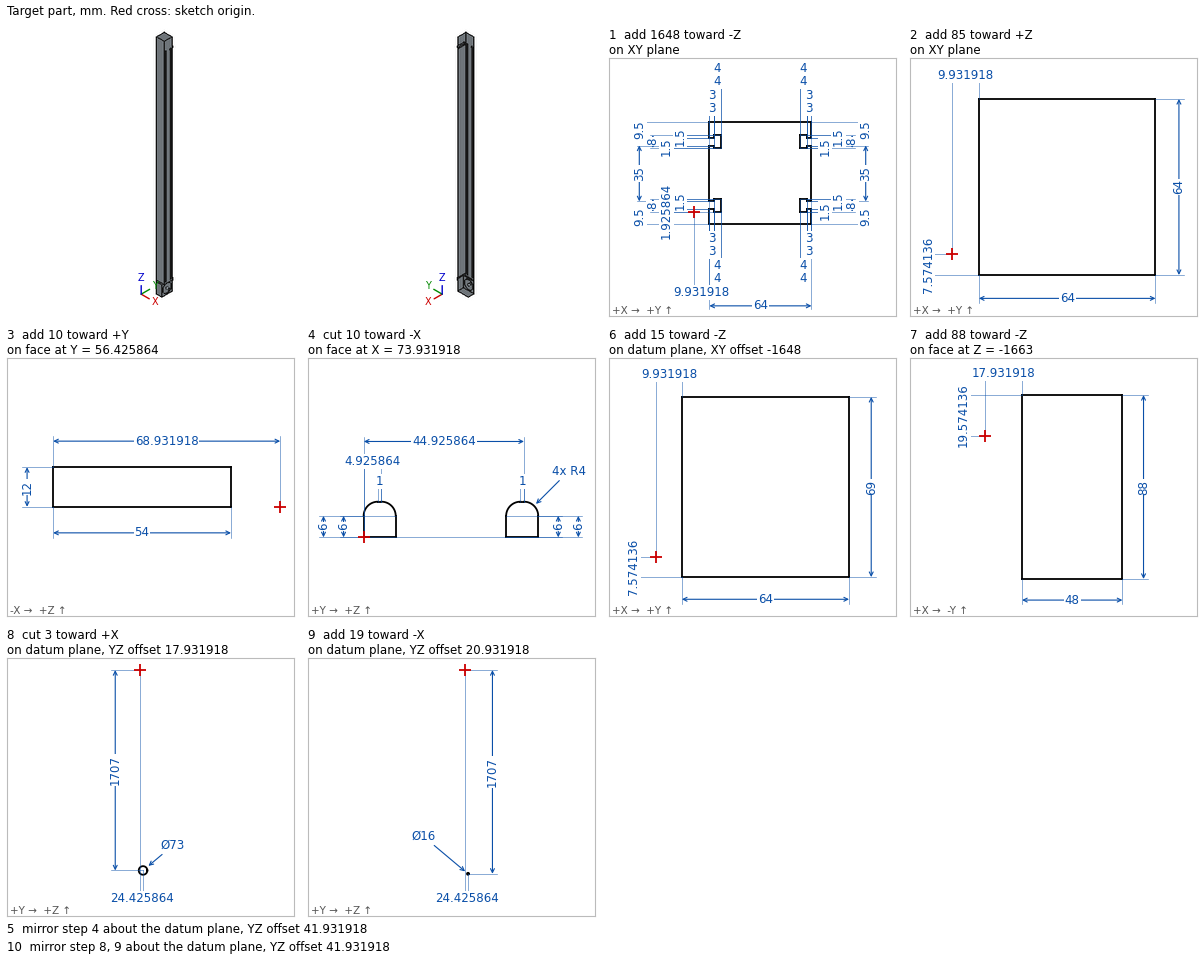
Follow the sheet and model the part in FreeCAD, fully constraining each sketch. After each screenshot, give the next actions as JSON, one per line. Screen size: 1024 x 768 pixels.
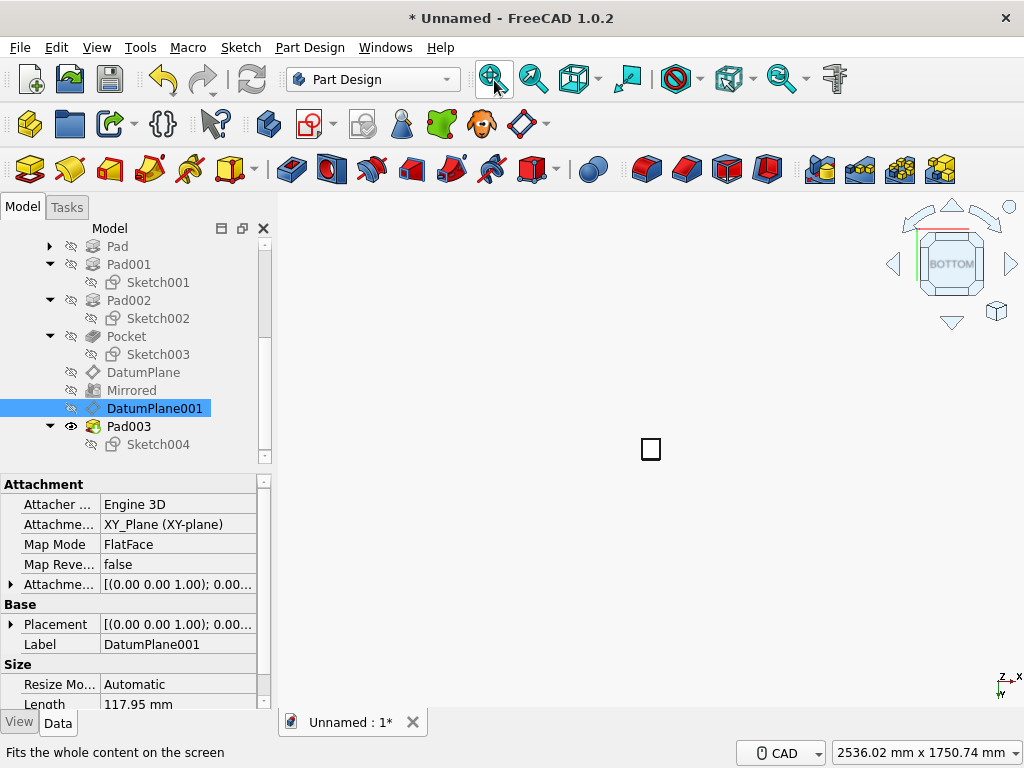
{"action": "left_click", "coordinate": [494, 80]}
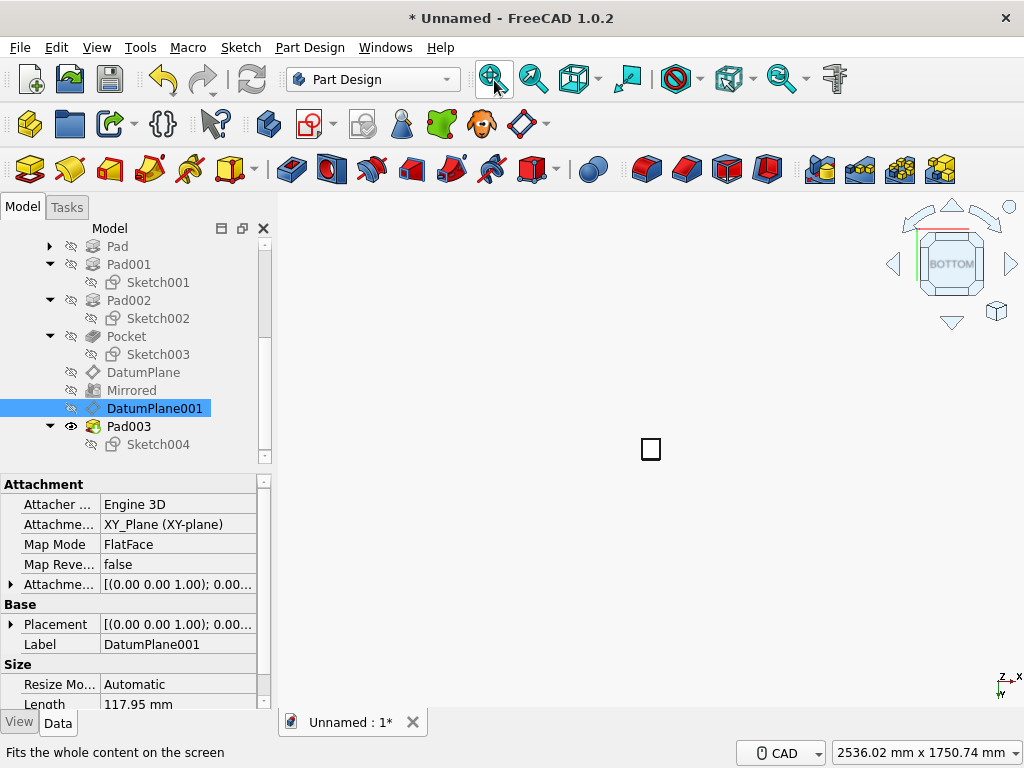
{"action": "left_click", "coordinate": [651, 448]}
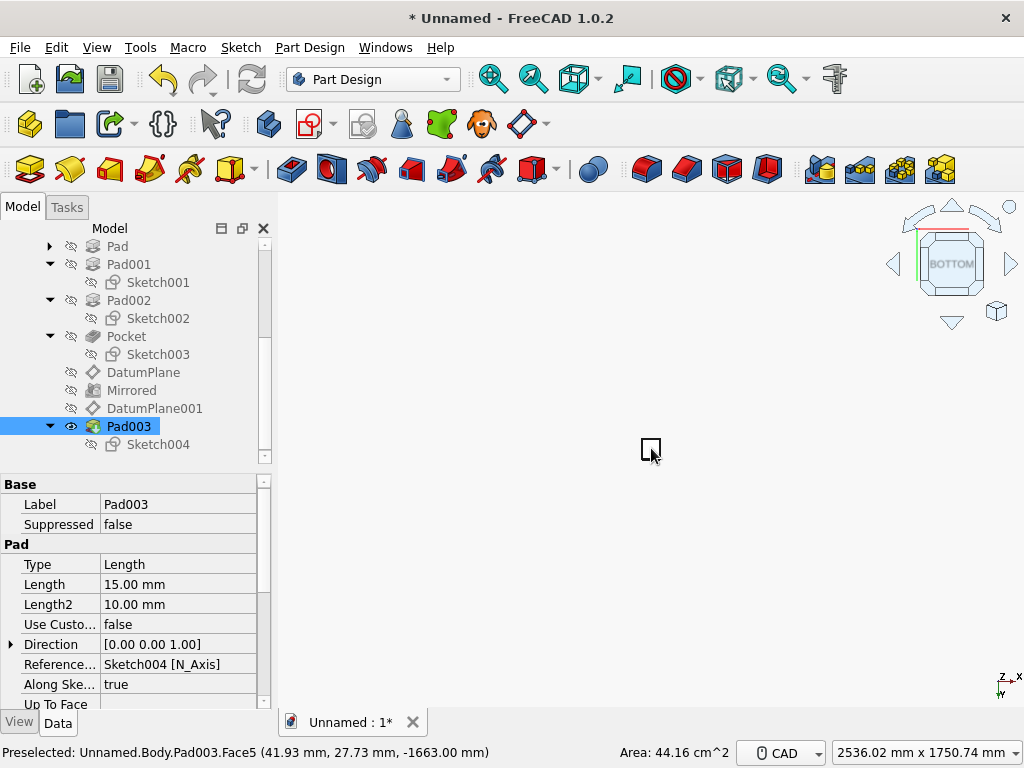
{"action": "left_click", "coordinate": [310, 124]}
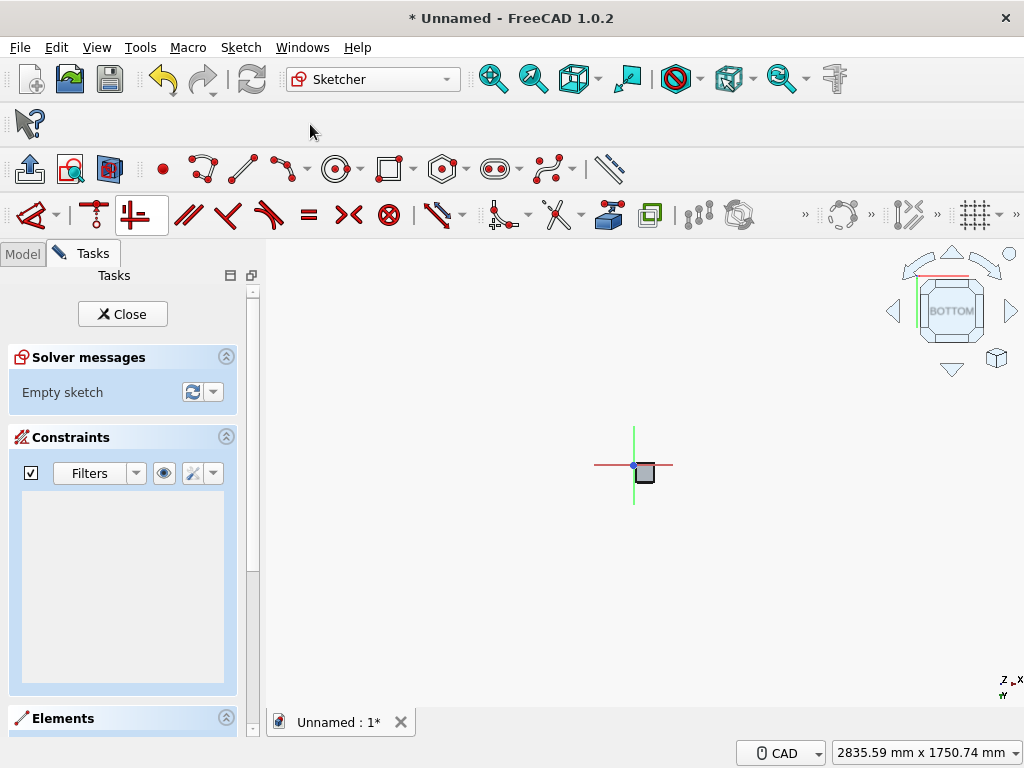
{"action": "scroll", "coordinate": [648, 472], "scroll_direction": "up", "scroll_amount": 13}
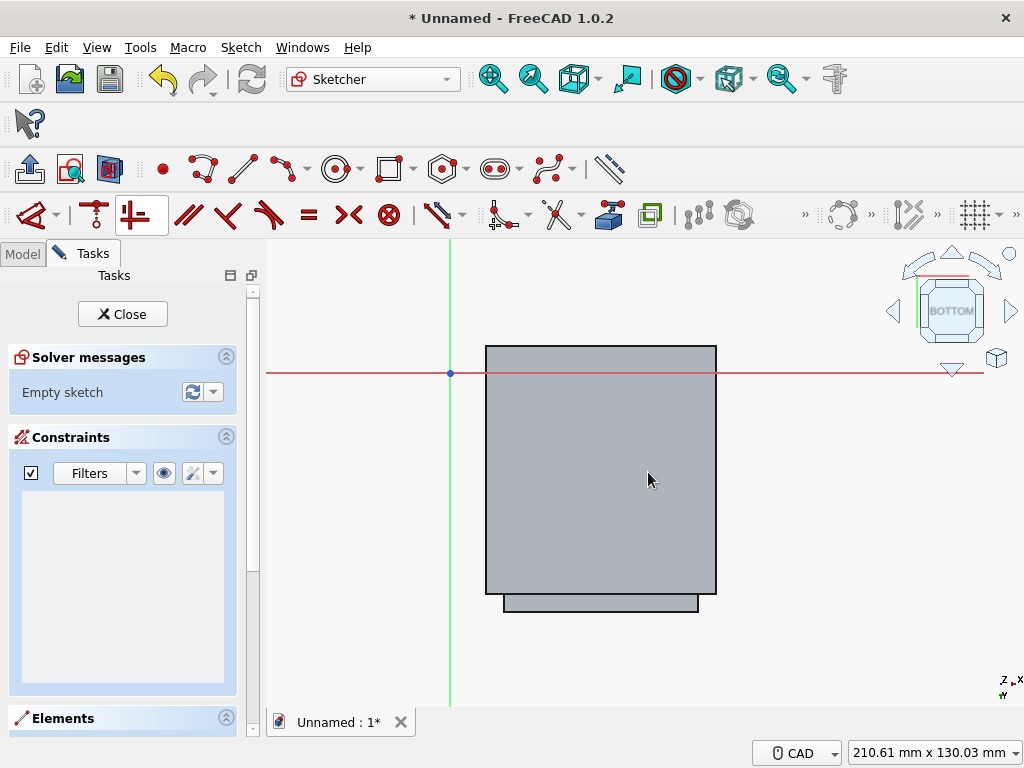
{"action": "left_click", "coordinate": [390, 170]}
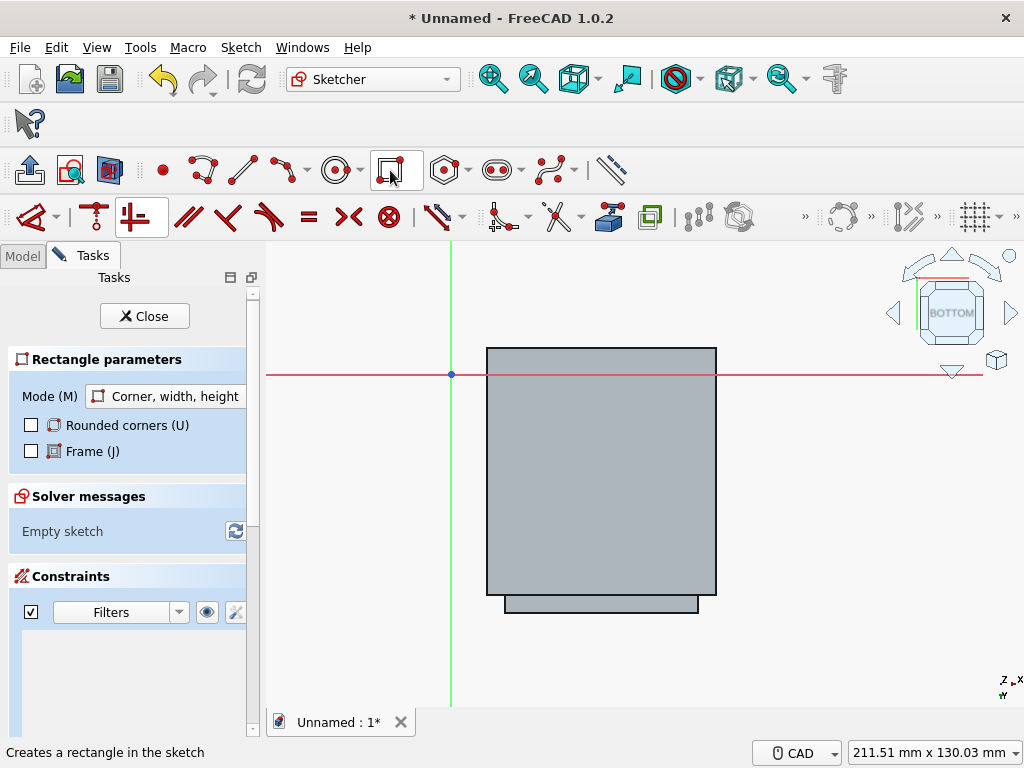
{"action": "left_click", "coordinate": [515, 305]}
{"action": "mouse_move", "coordinate": [688, 620]}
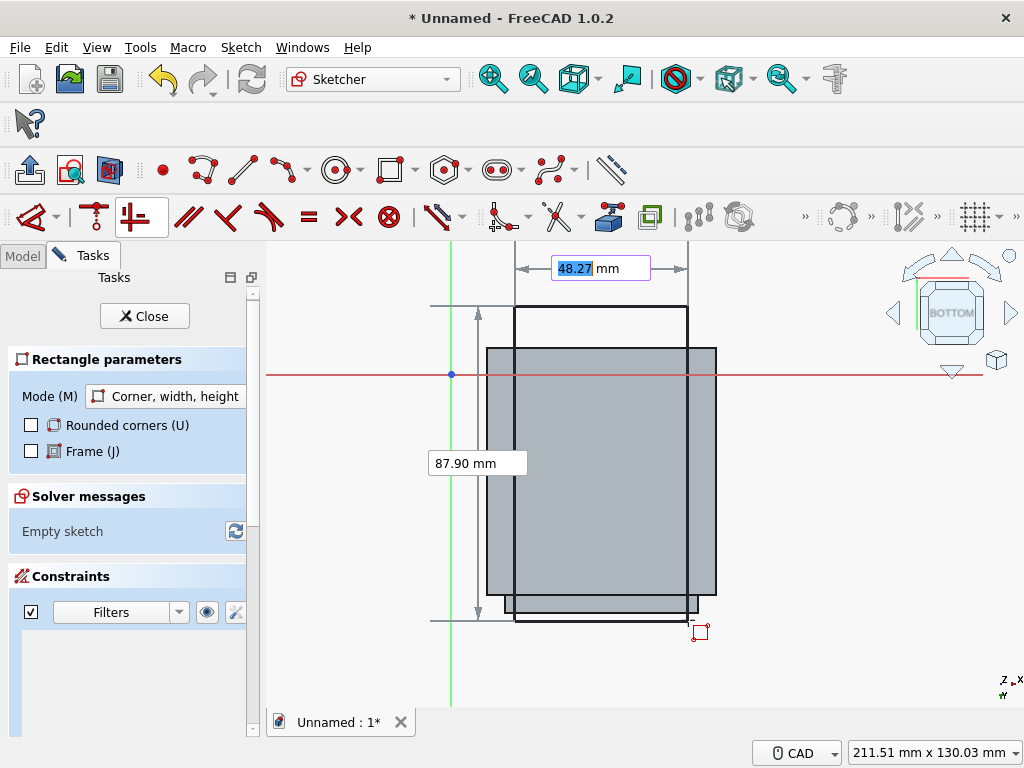
{"action": "type", "text": "48"}
{"action": "key", "text": "Tab"}
{"action": "type", "text": "88"}
{"action": "key", "text": "Return"}
{"action": "key", "text": "Escape"}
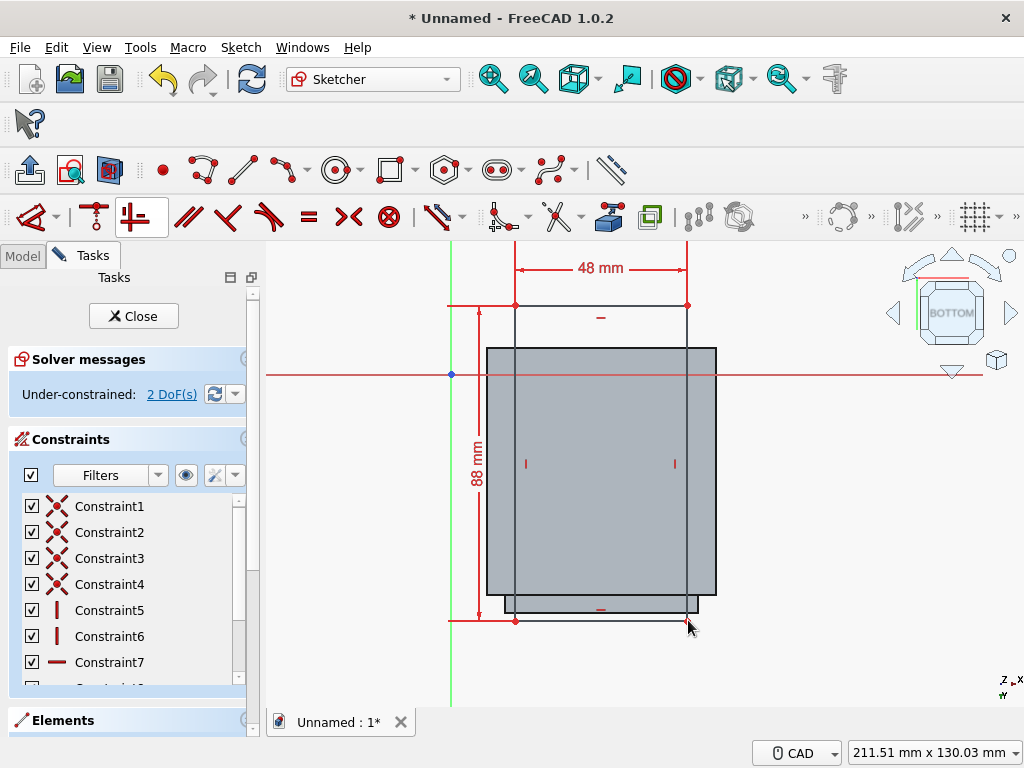
{"action": "left_click", "coordinate": [32, 218]}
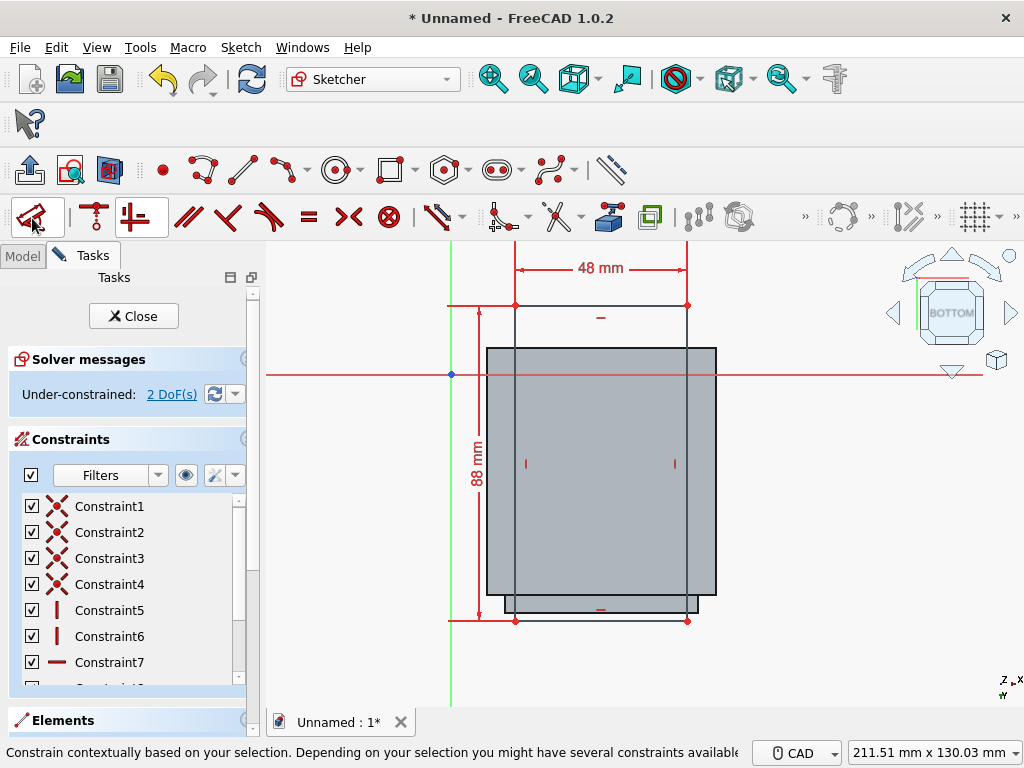
{"action": "left_click", "coordinate": [515, 306]}
{"action": "left_click", "coordinate": [483, 272]}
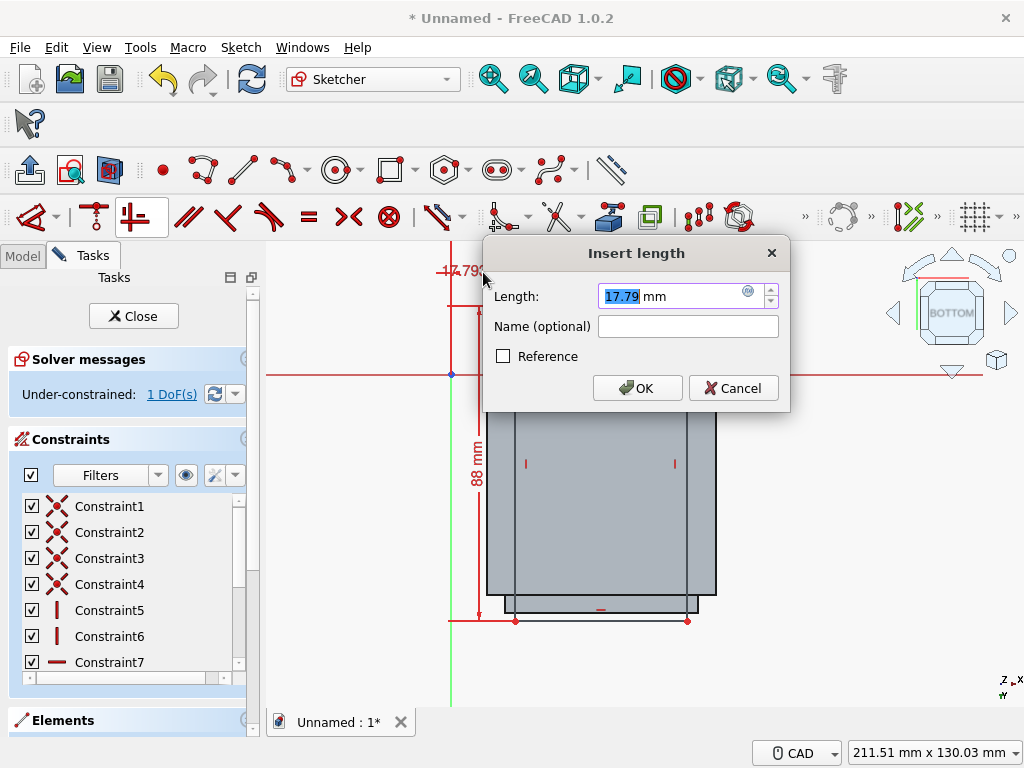
{"action": "type", "text": "17.931918"}
{"action": "key", "text": "Return"}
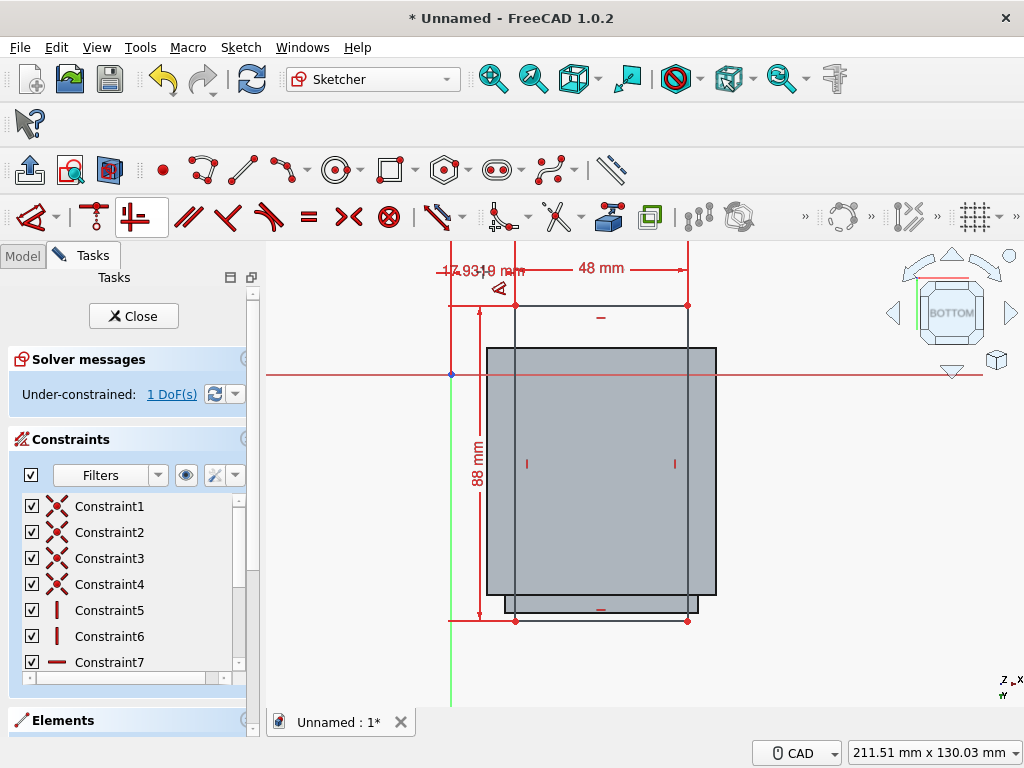
{"action": "left_click", "coordinate": [515, 306]}
{"action": "left_click", "coordinate": [417, 340]}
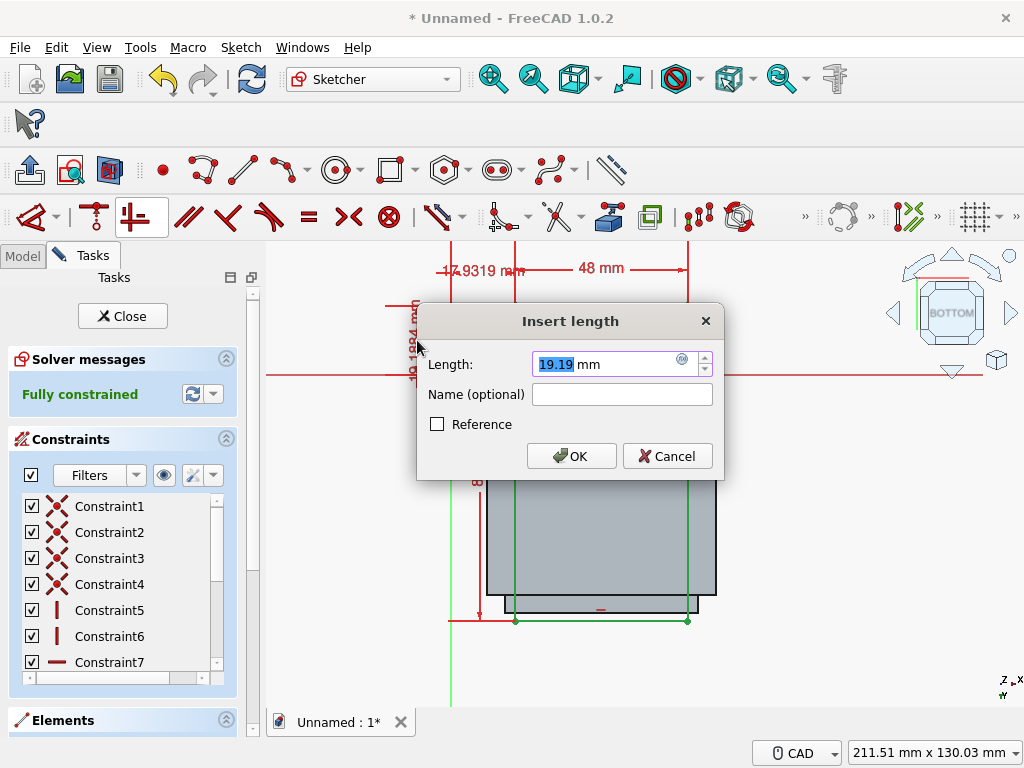
{"action": "type", "text": "19.574136"}
{"action": "key", "text": "Return"}
{"action": "key", "text": "Escape"}